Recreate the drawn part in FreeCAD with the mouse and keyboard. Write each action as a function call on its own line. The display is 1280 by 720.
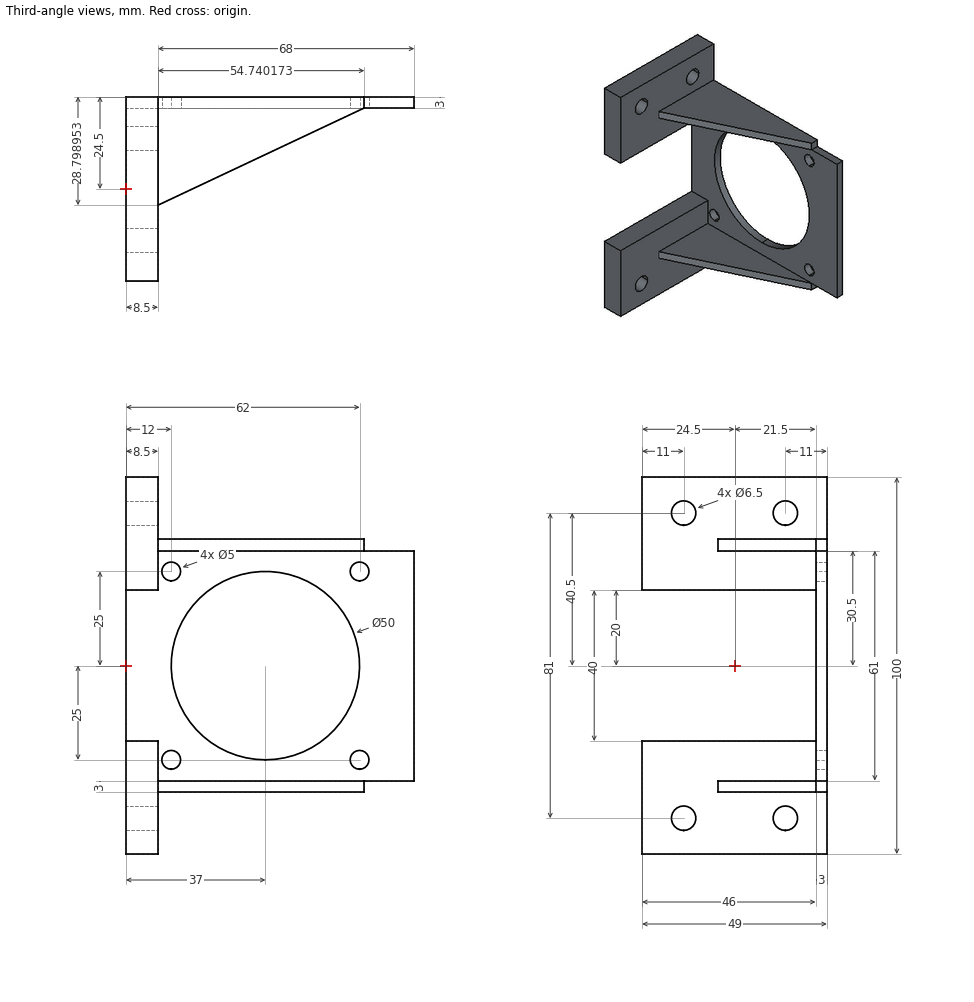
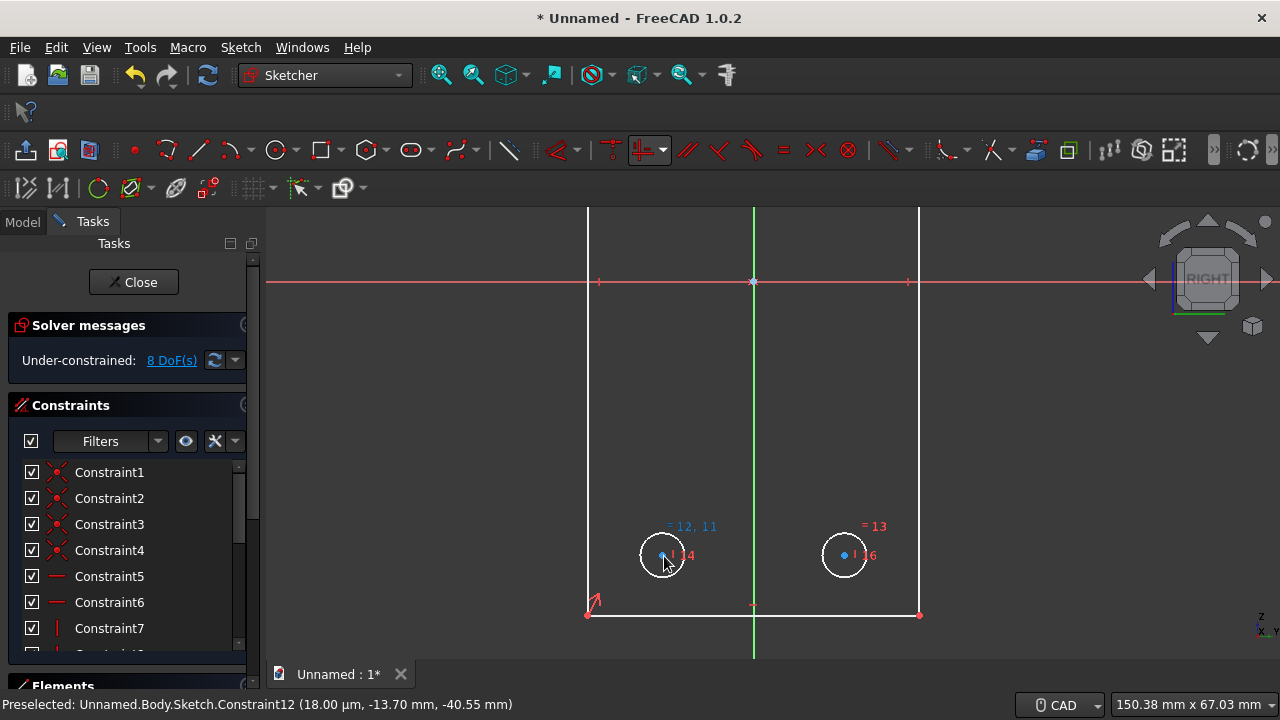
click(662, 555)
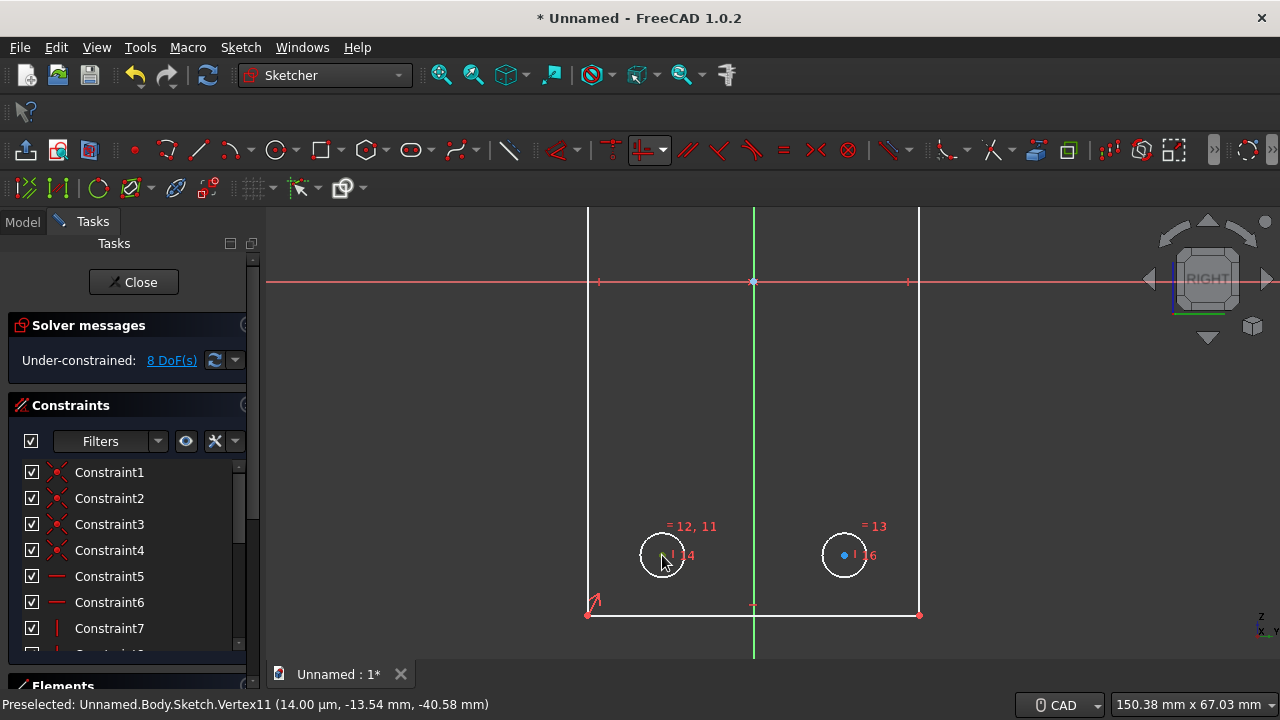
click(844, 555)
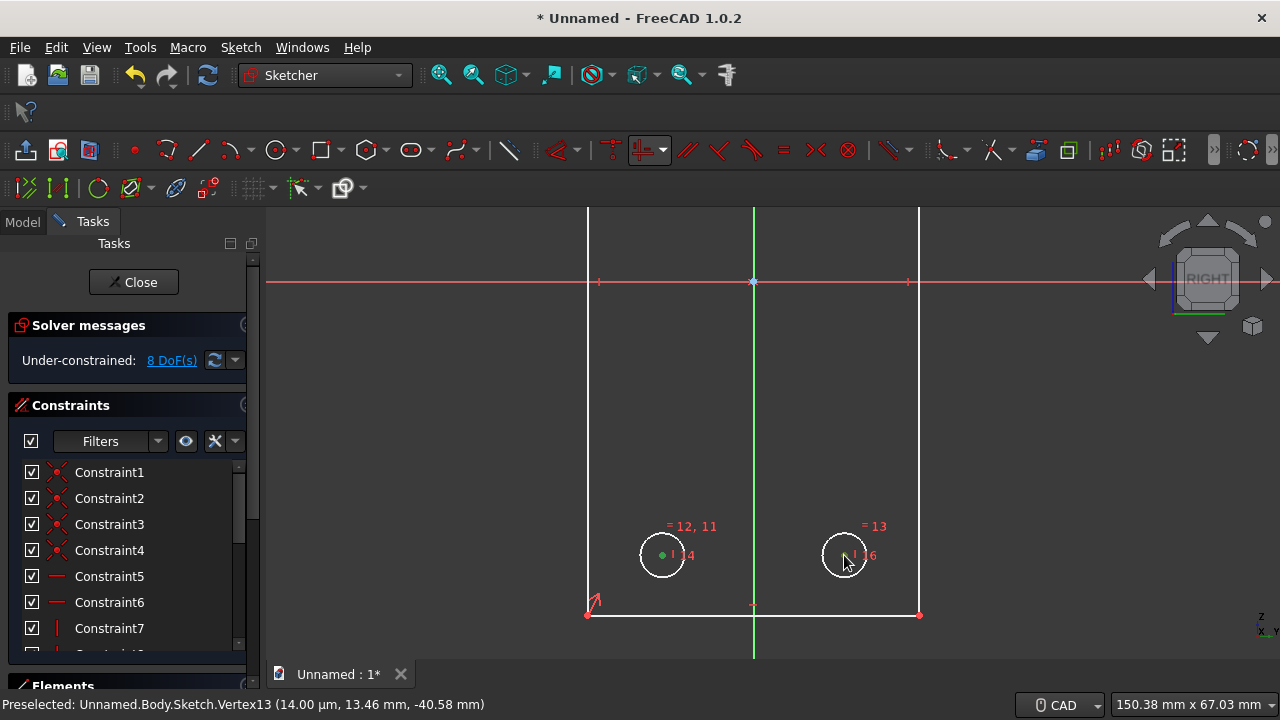
click(666, 150)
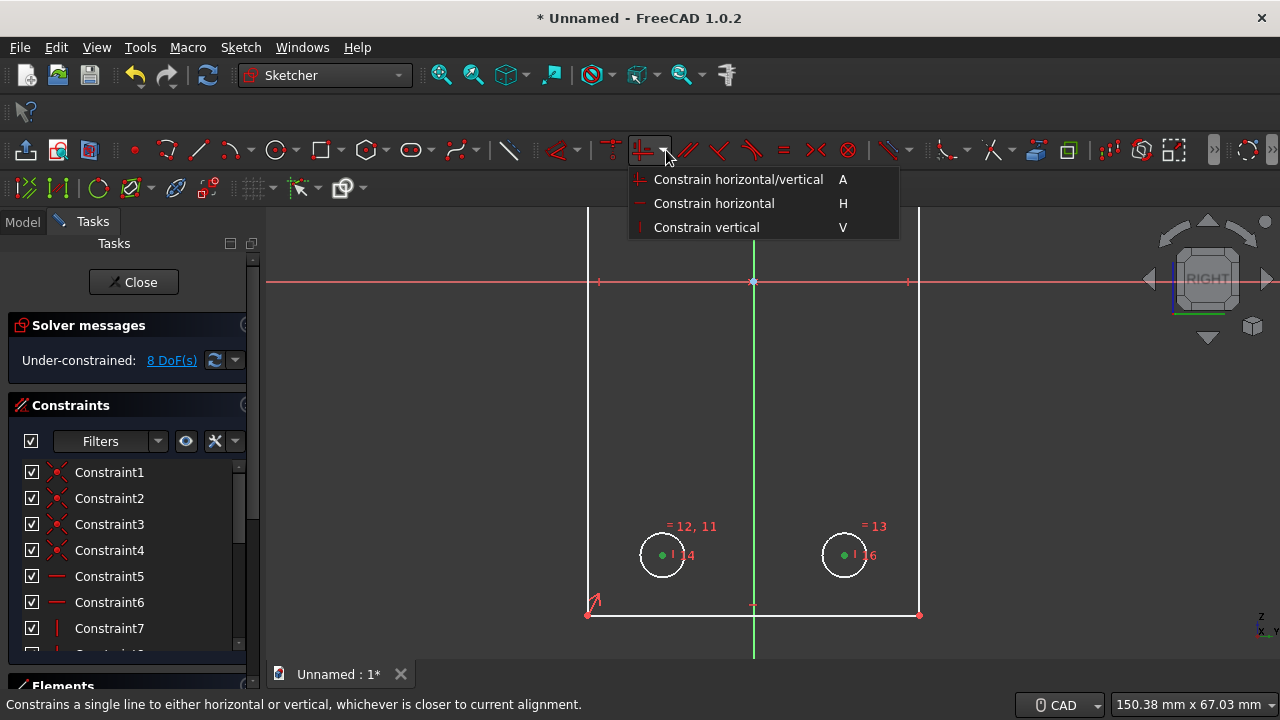
click(764, 203)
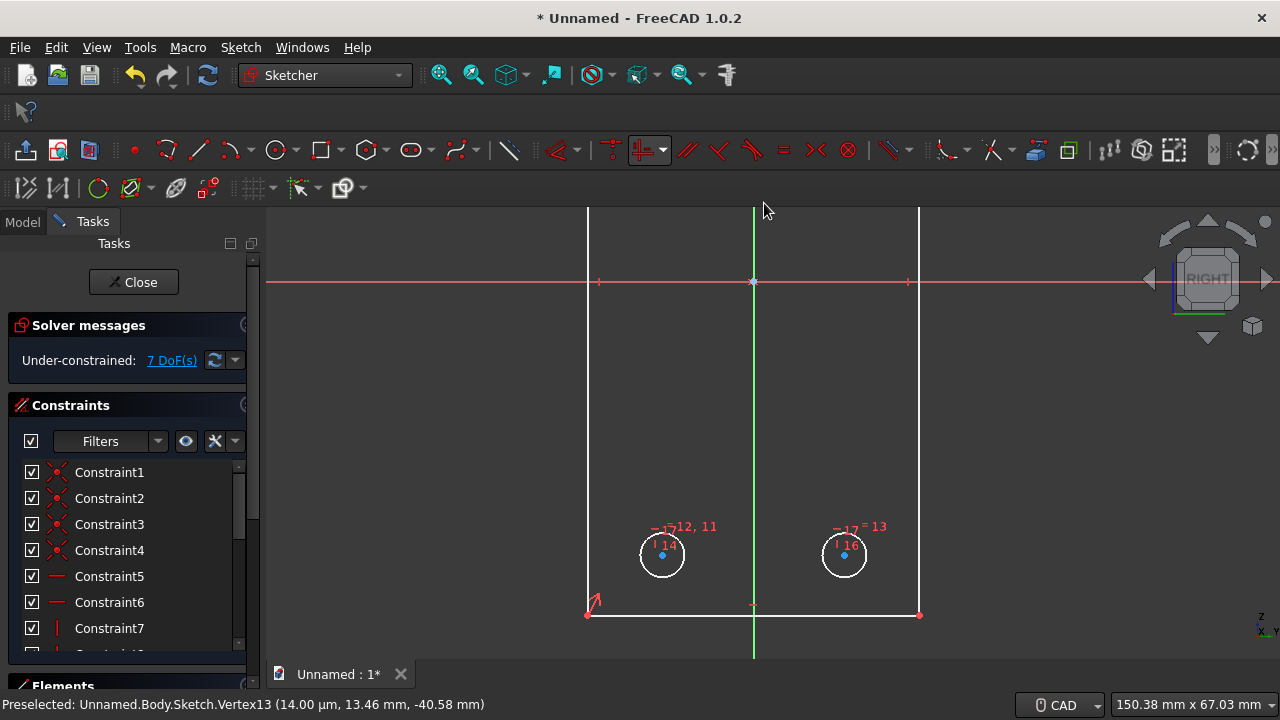
click(556, 150)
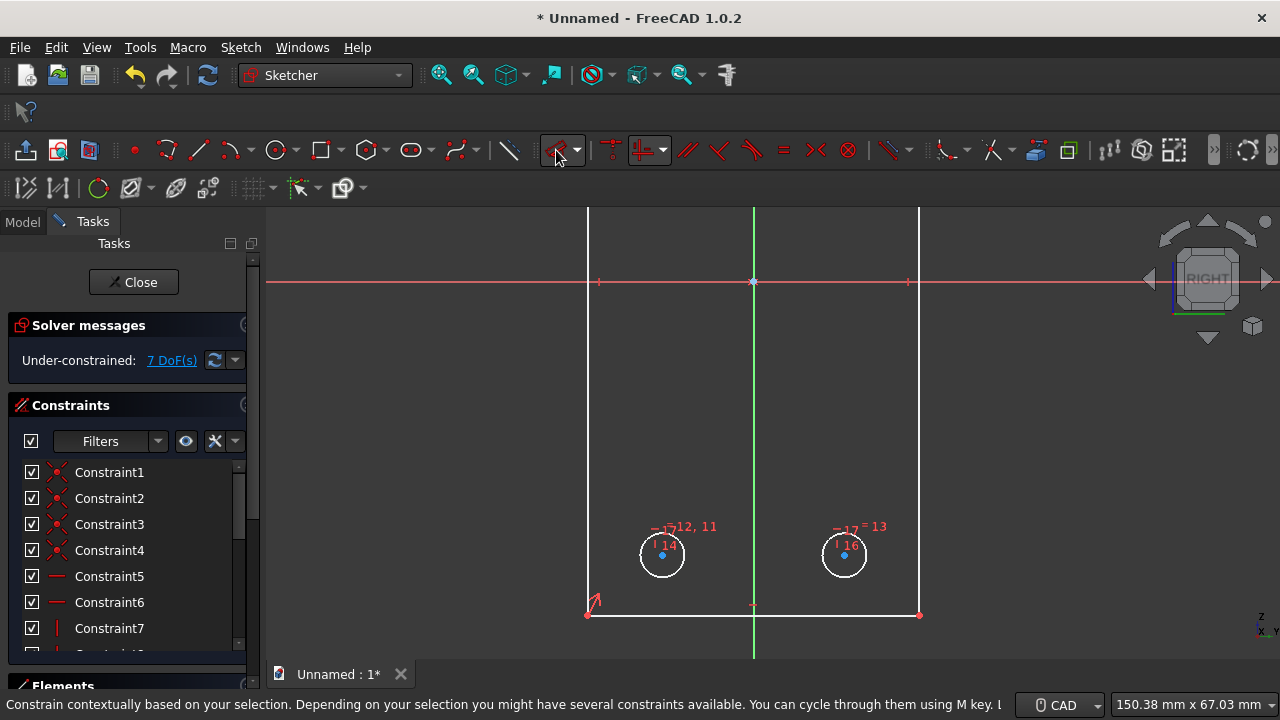
scroll(664, 557, down, 4)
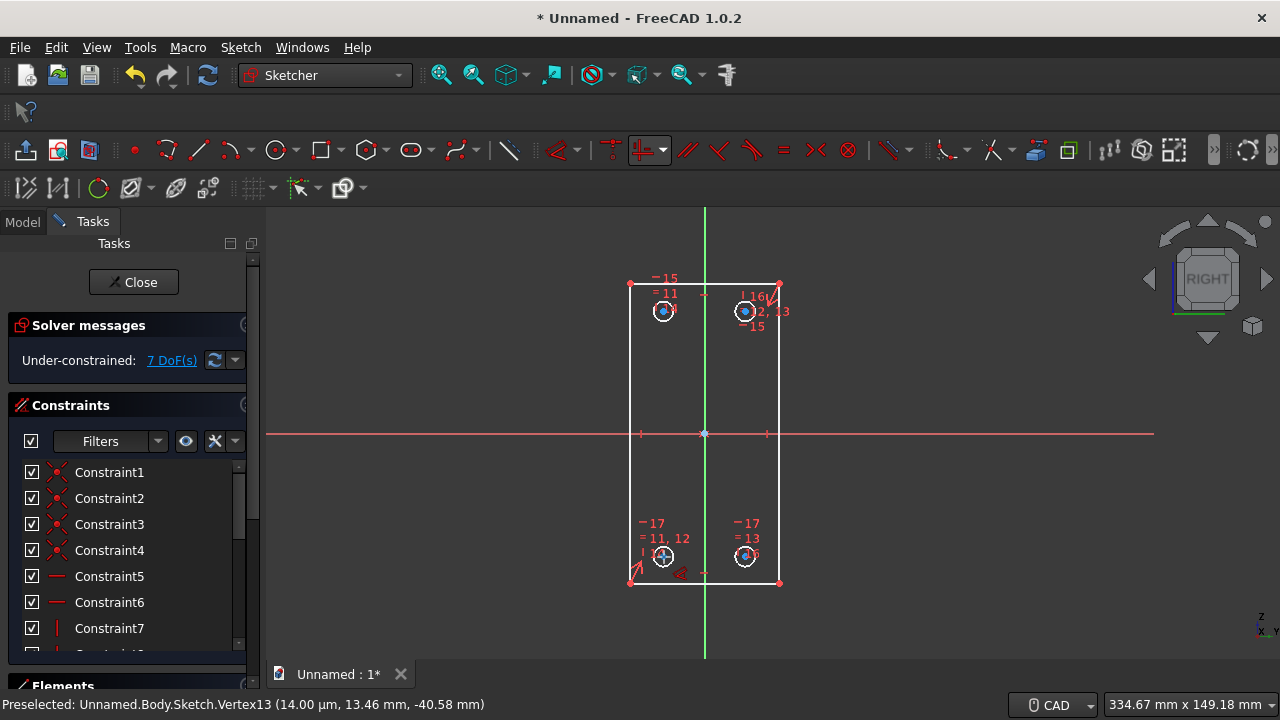
scroll(670, 304, up, 4)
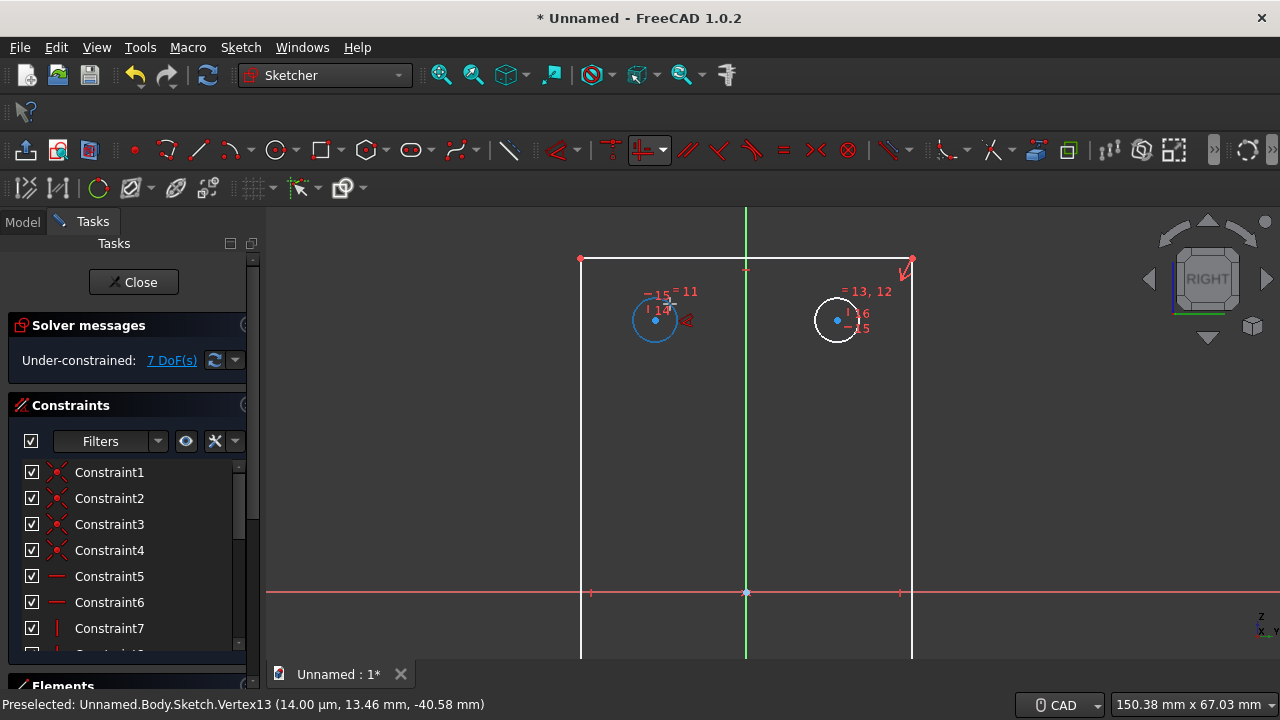
click(671, 305)
click(694, 283)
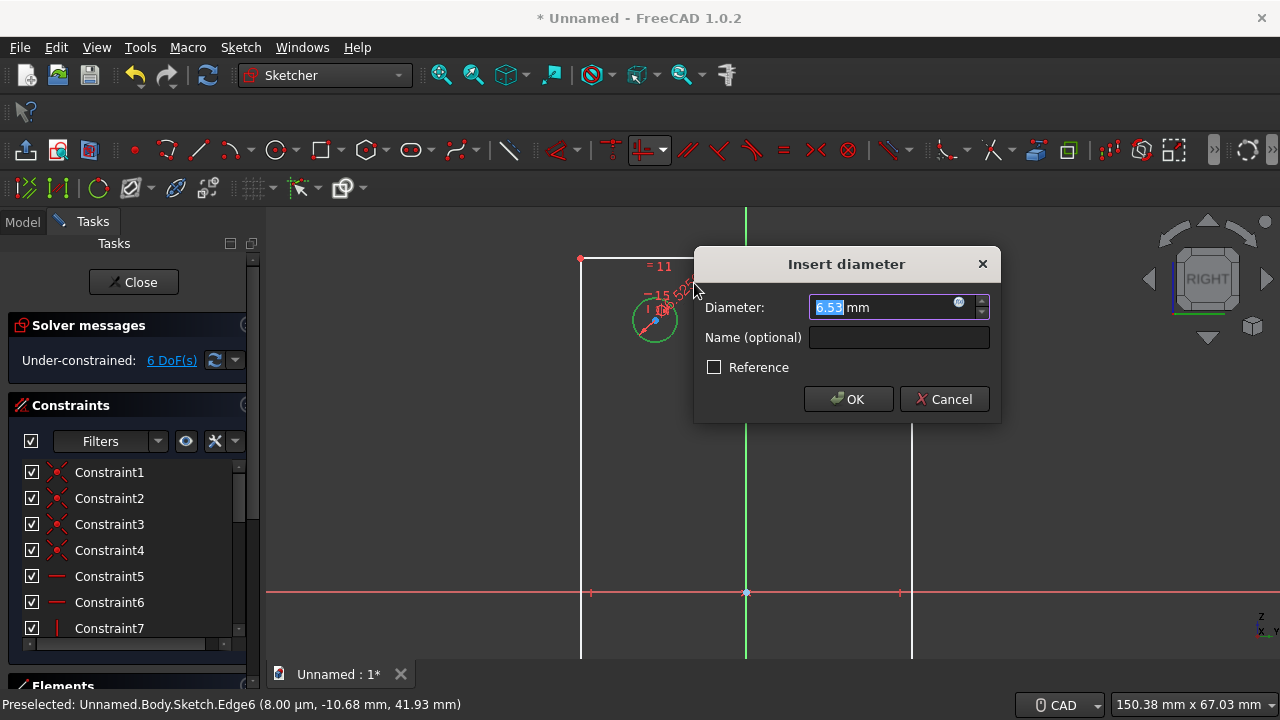
text(6.5)
key(Return)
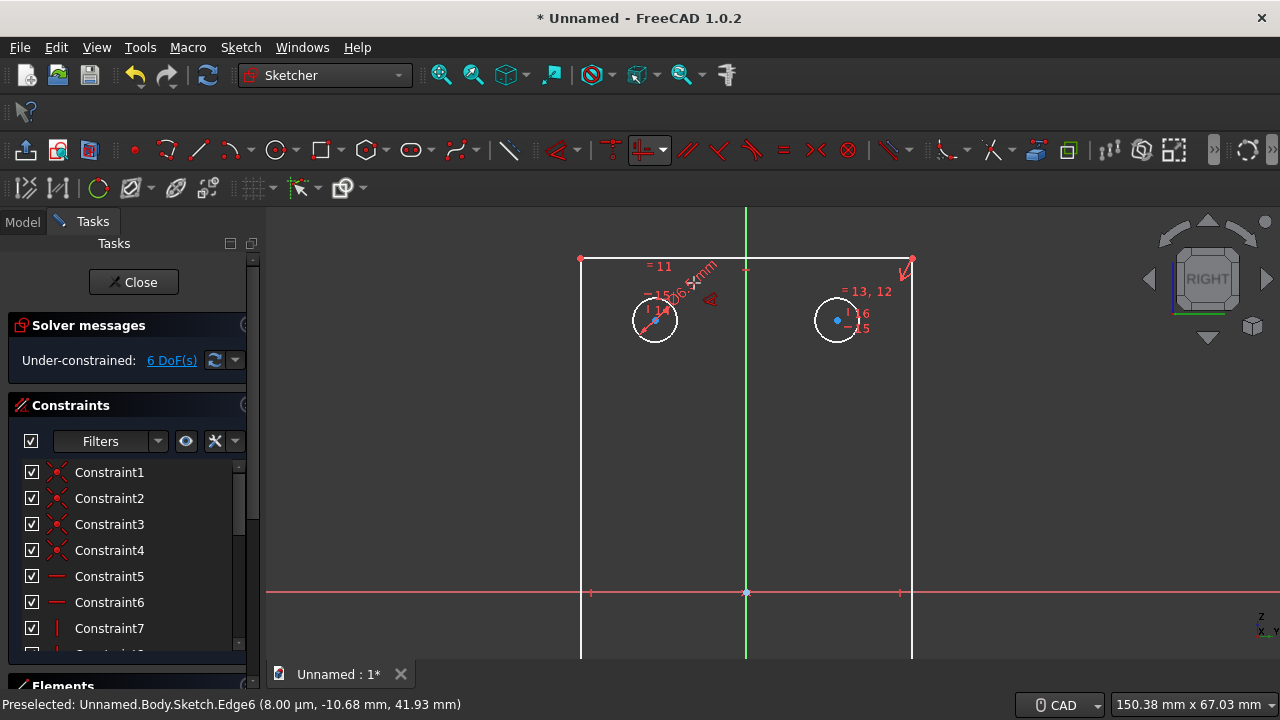
scroll(670, 303, down, 4)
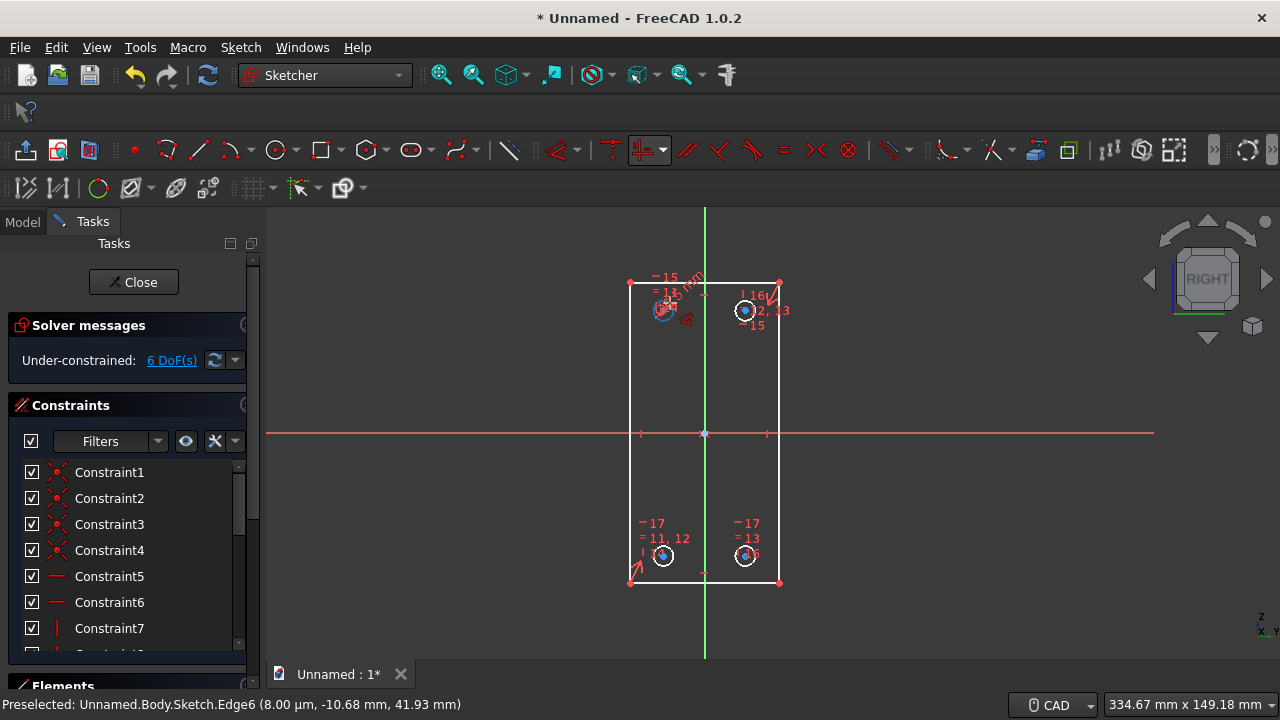
click(675, 583)
click(670, 617)